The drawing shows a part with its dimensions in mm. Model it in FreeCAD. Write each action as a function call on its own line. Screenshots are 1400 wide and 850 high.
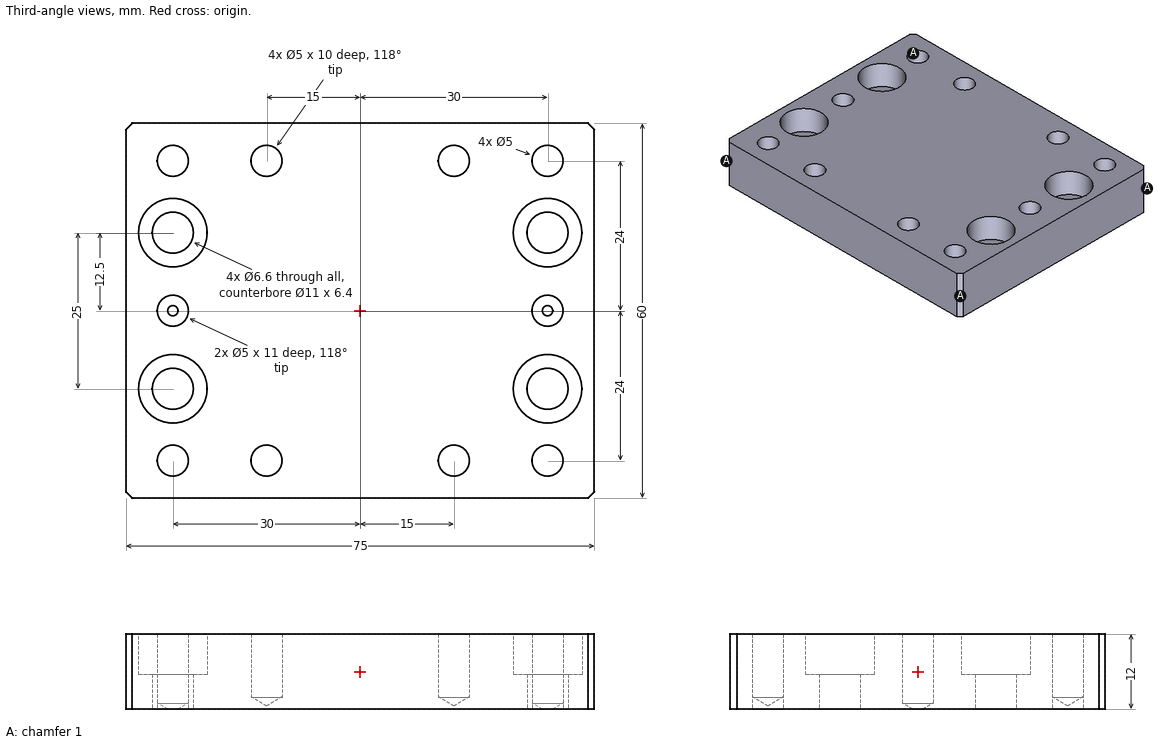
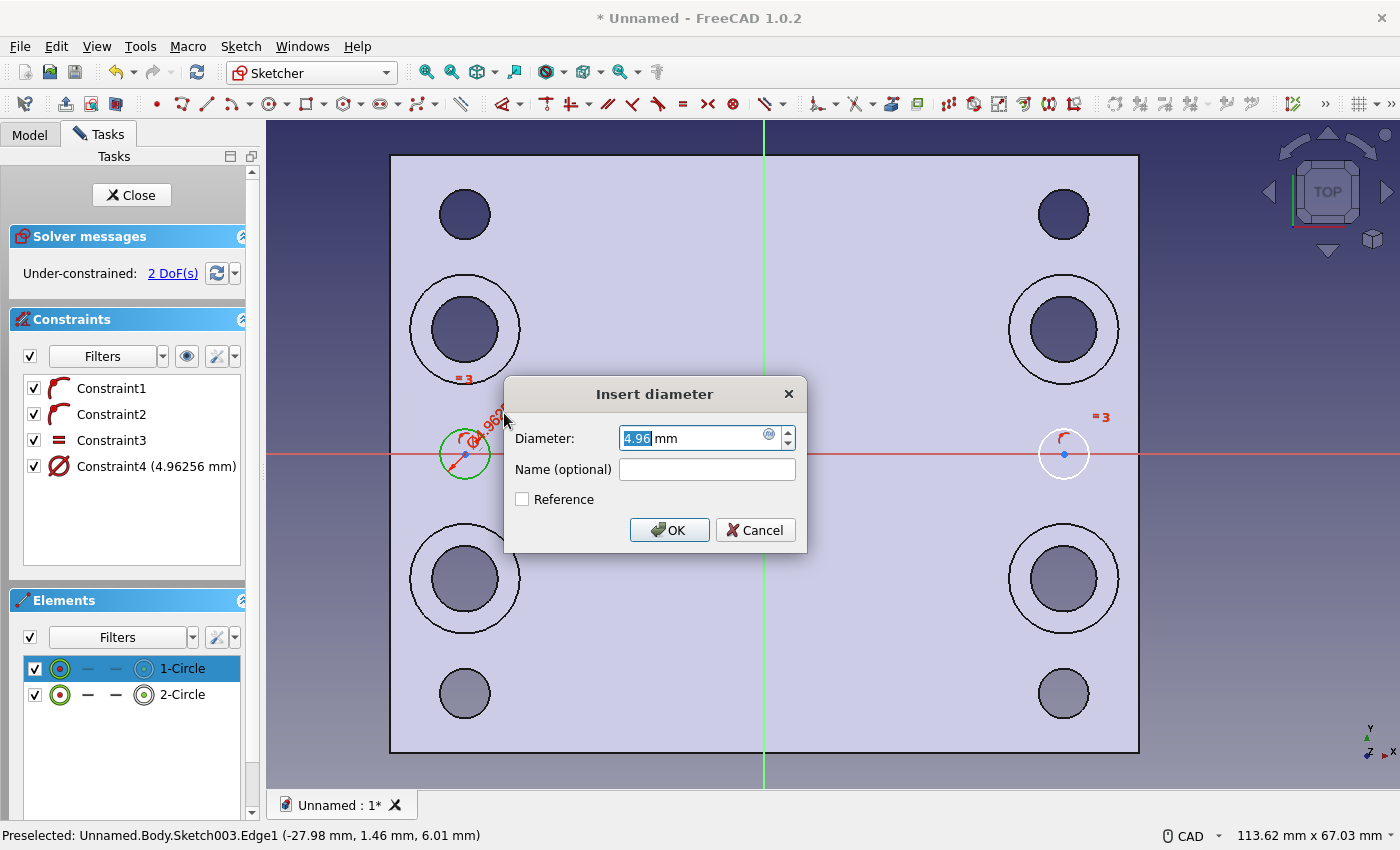
text(5)
key(Return)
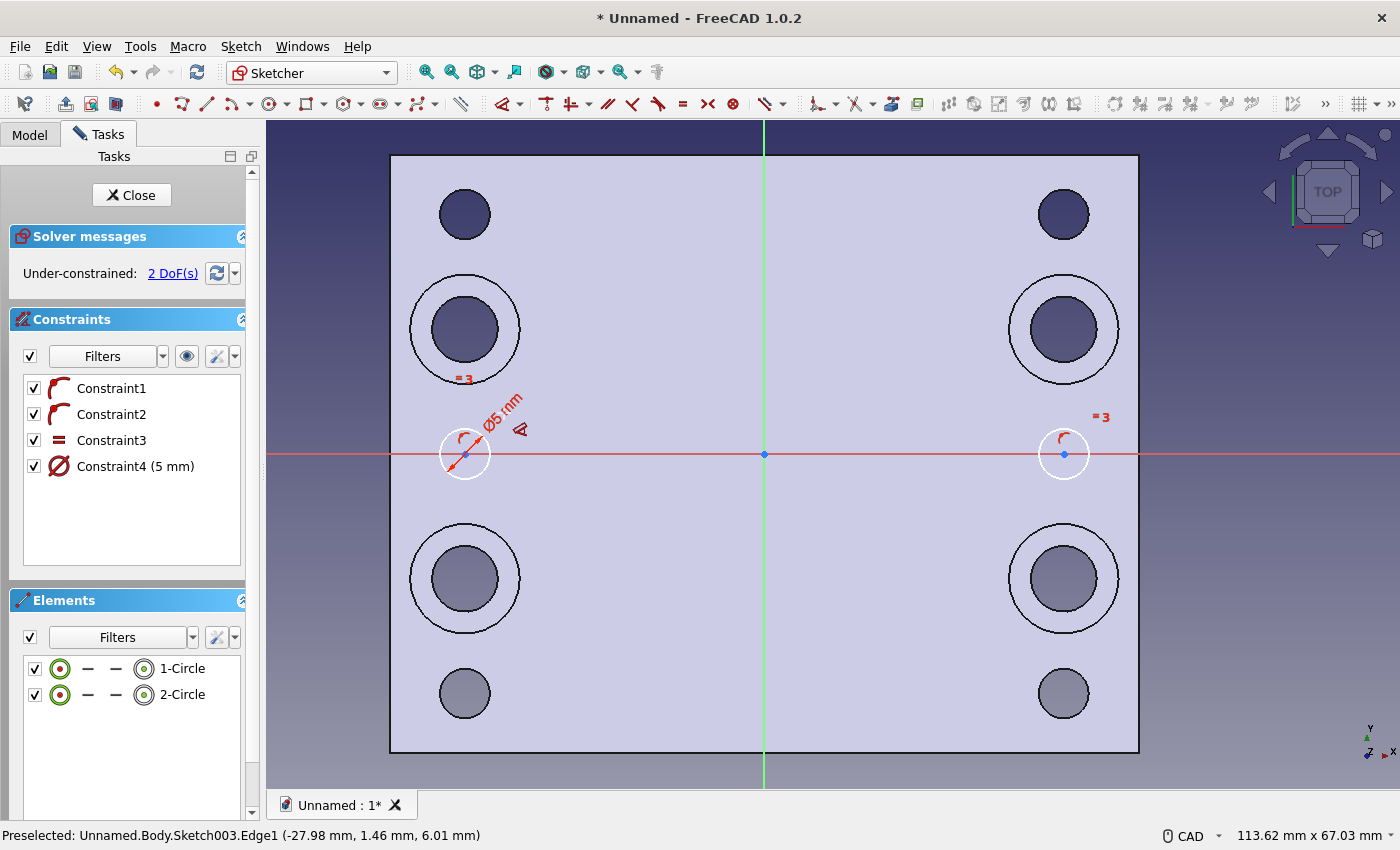
click(465, 454)
click(615, 488)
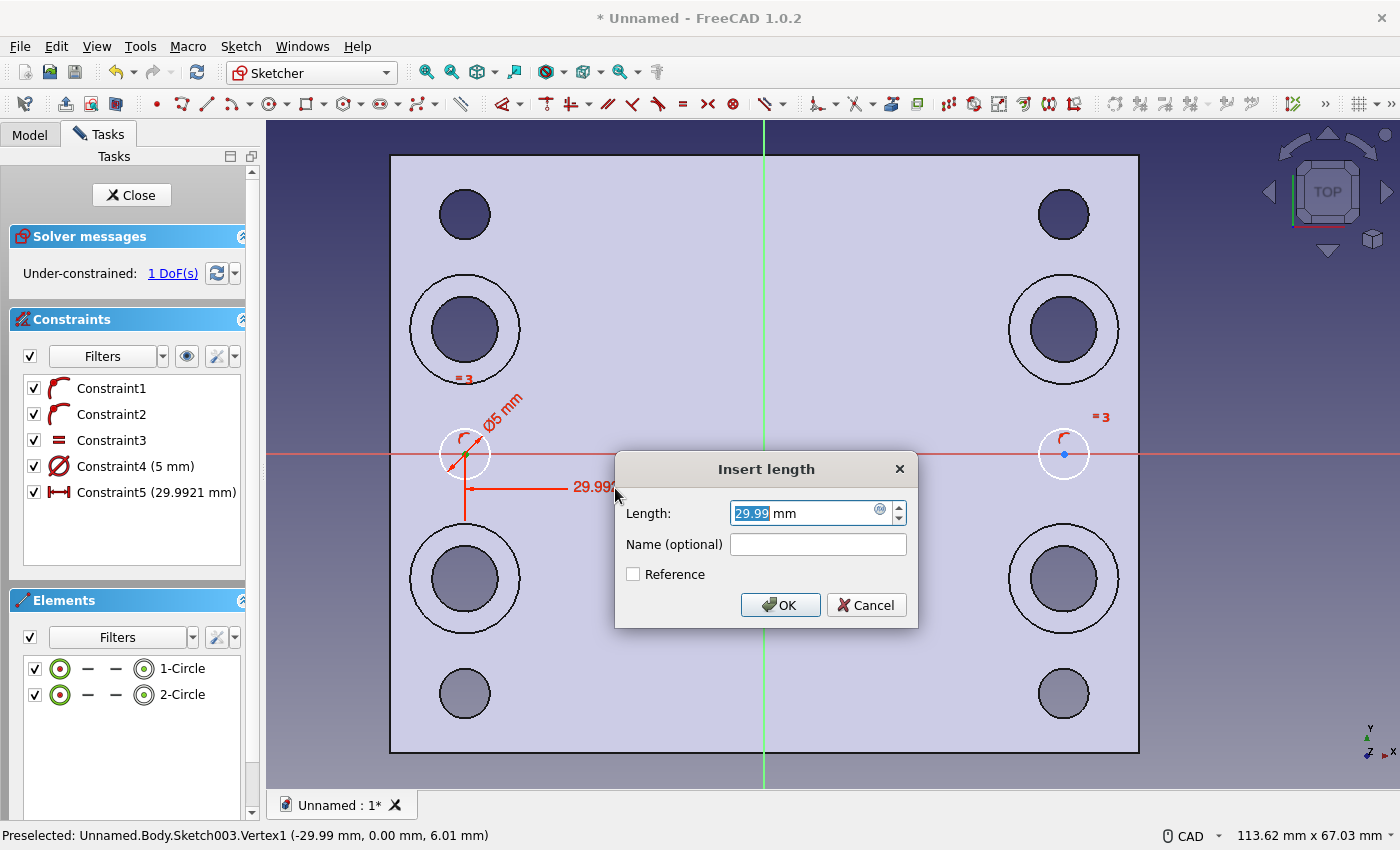
text(30)
key(Return)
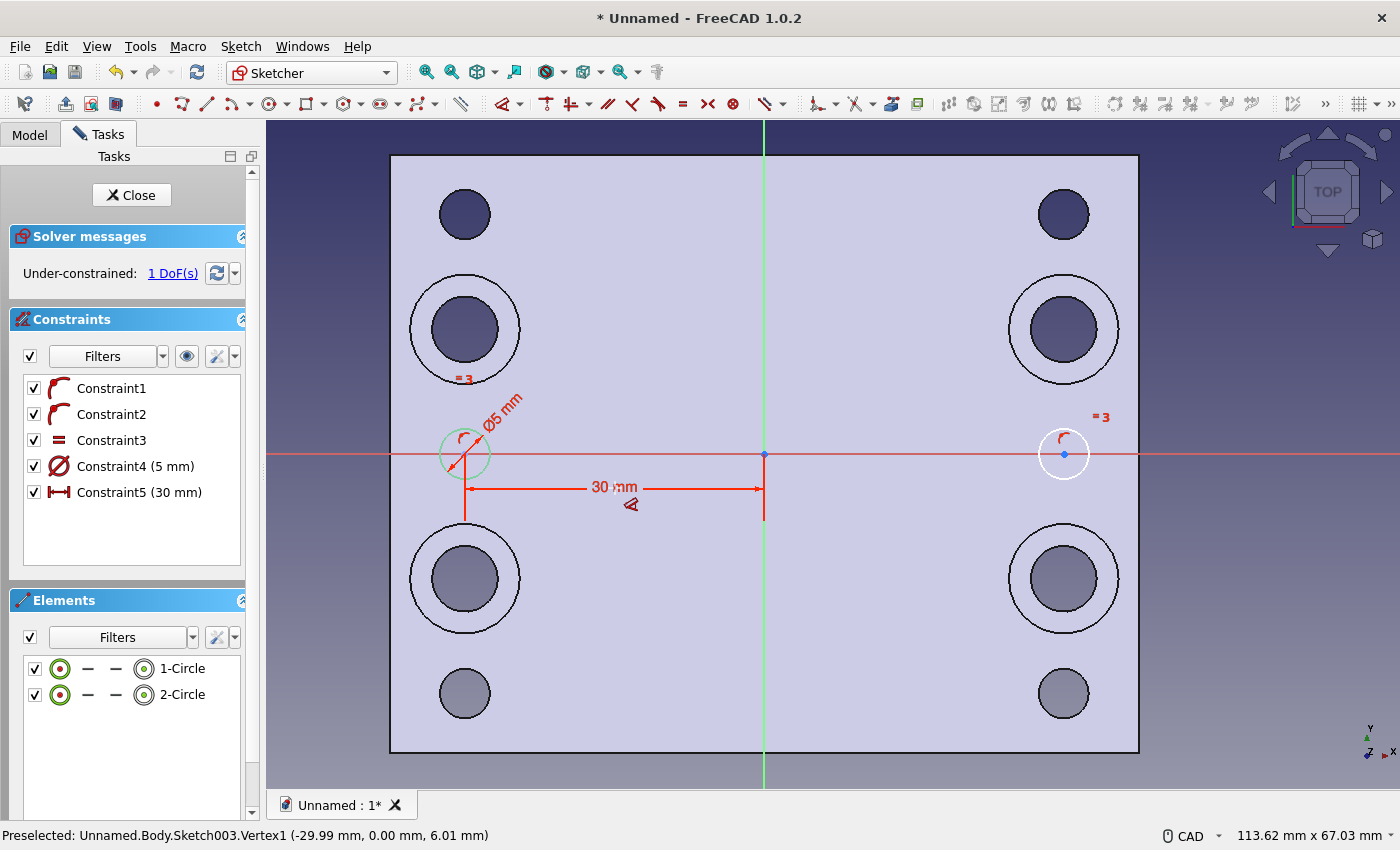
click(1064, 454)
click(914, 488)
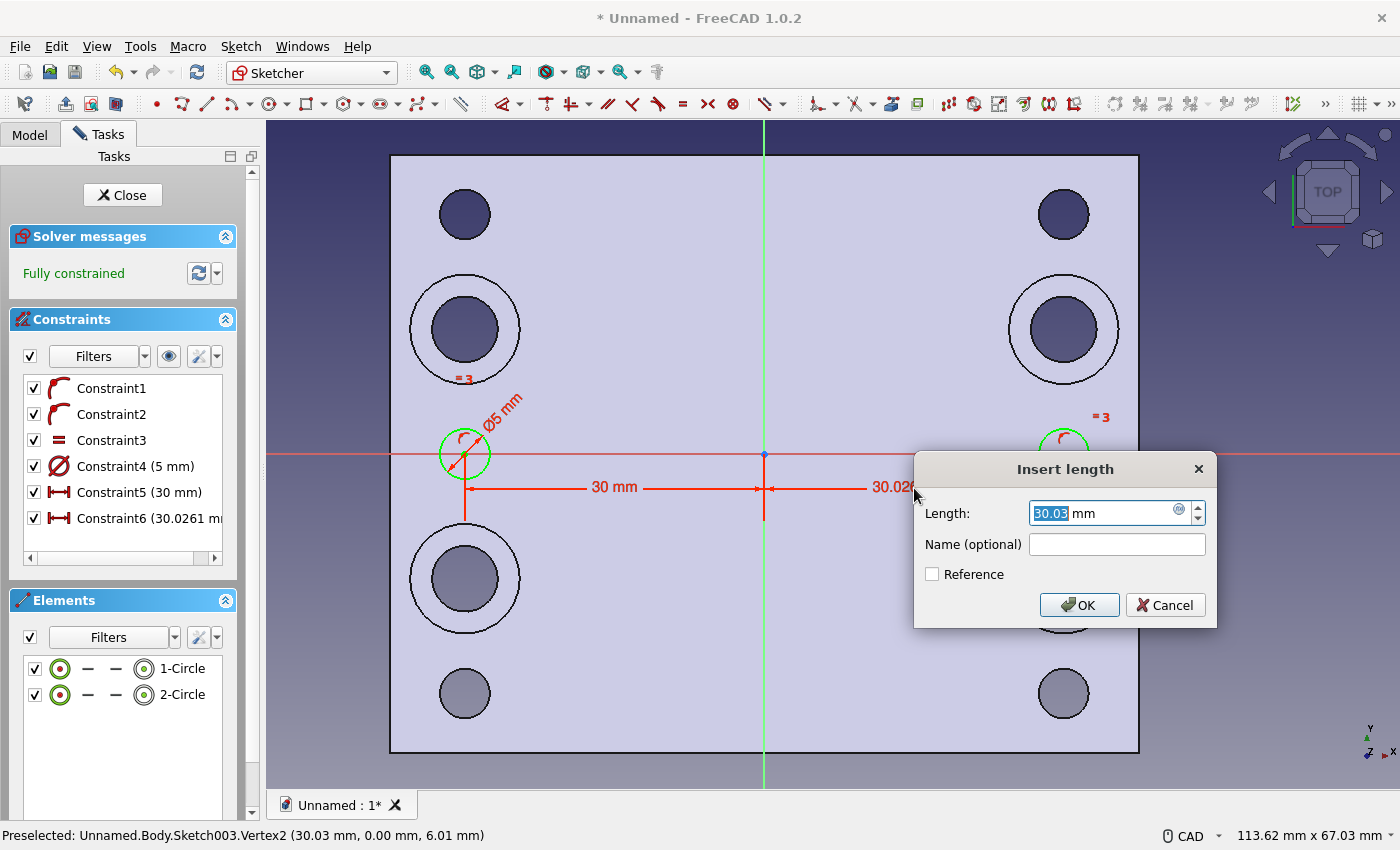
text(30)
key(Return)
key(Escape)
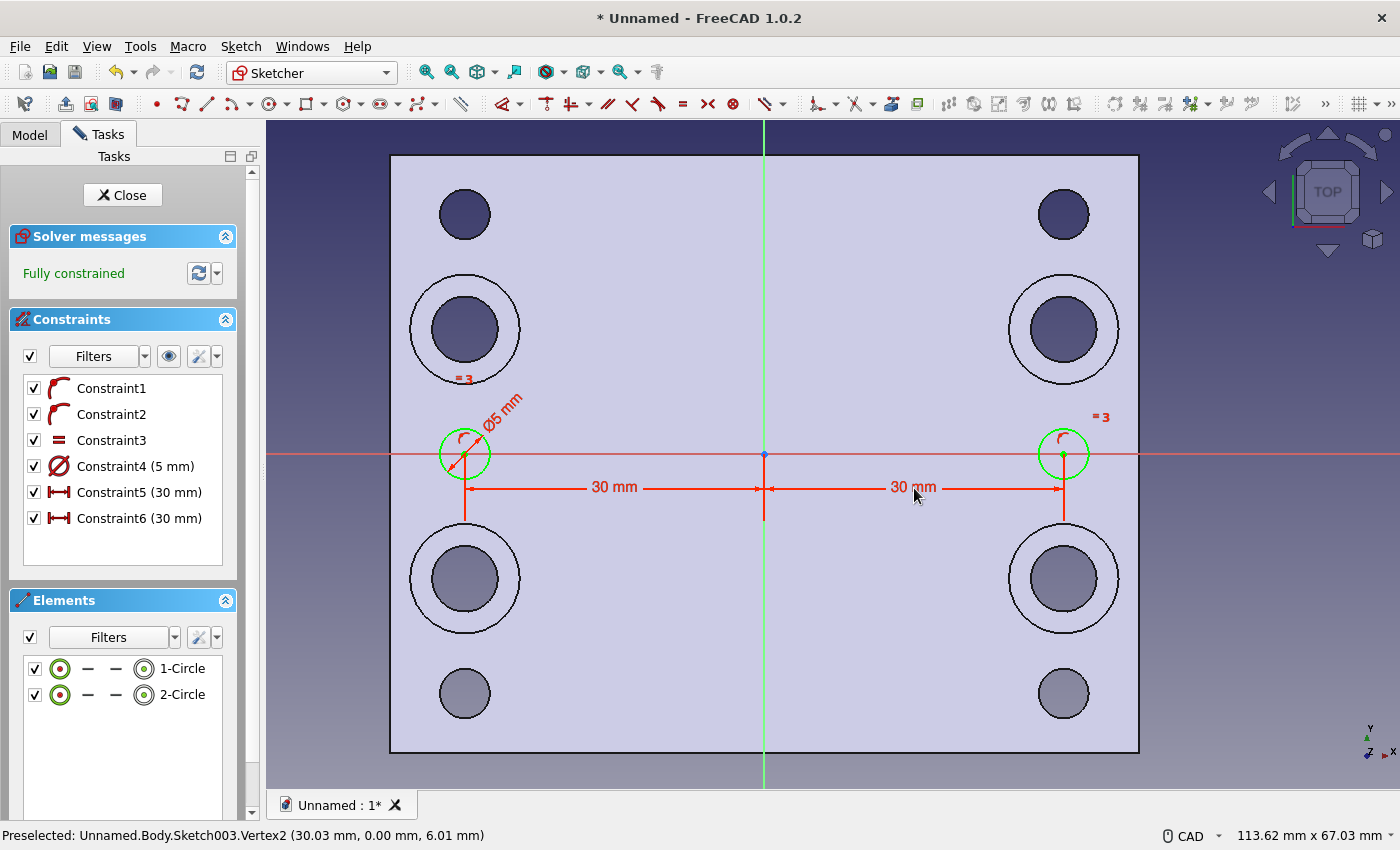
click(123, 195)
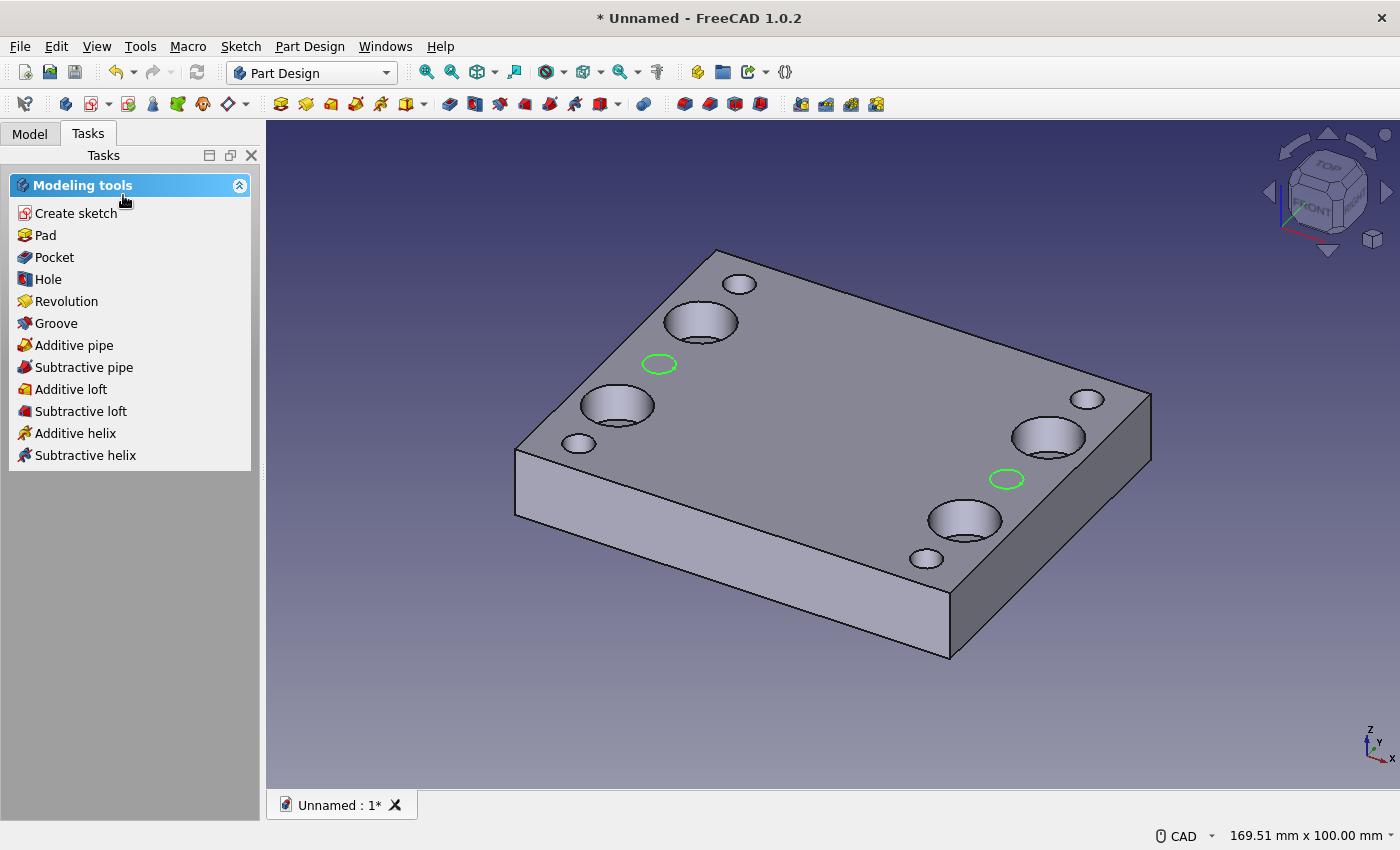
click(475, 104)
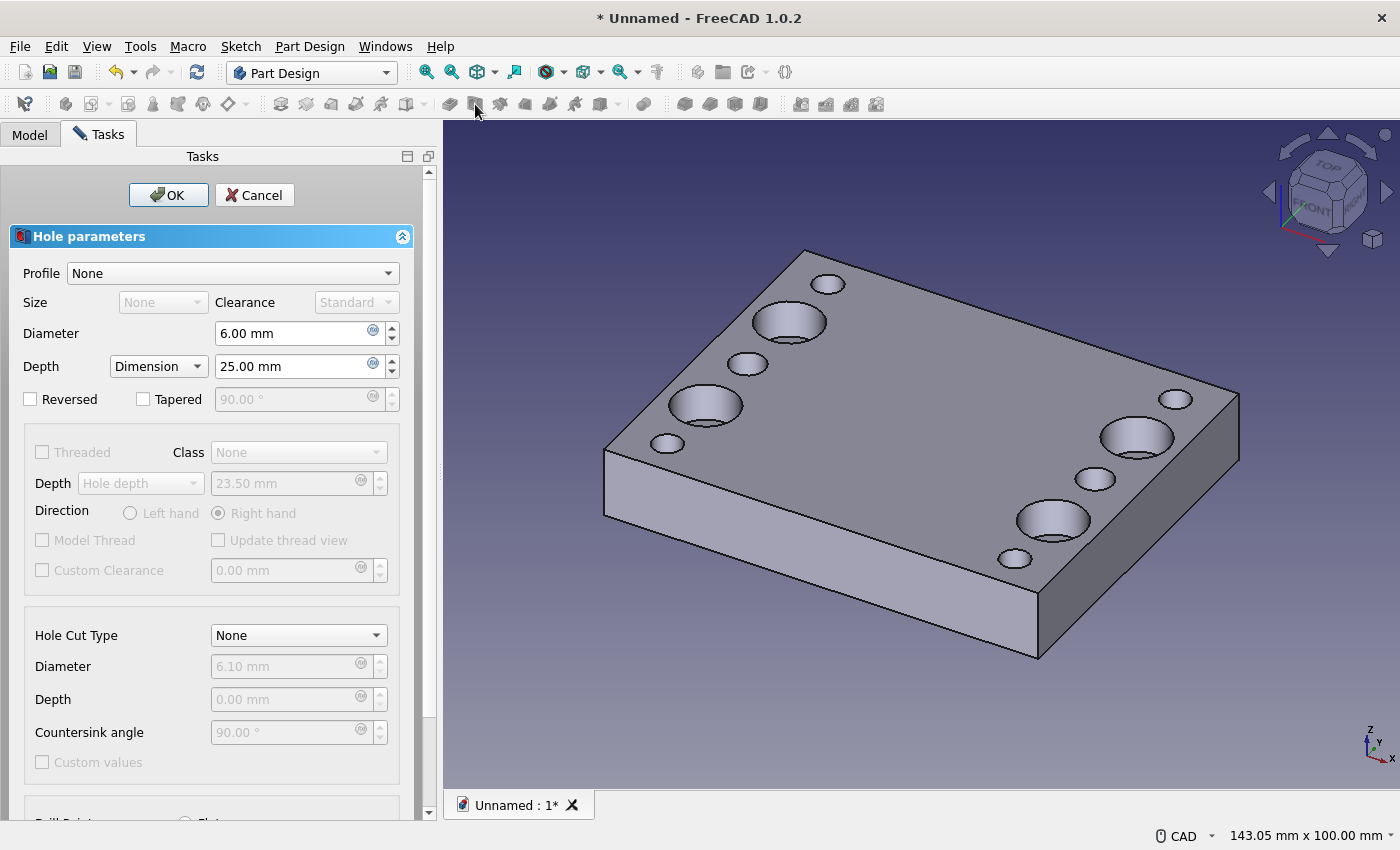
triple_click(300, 334)